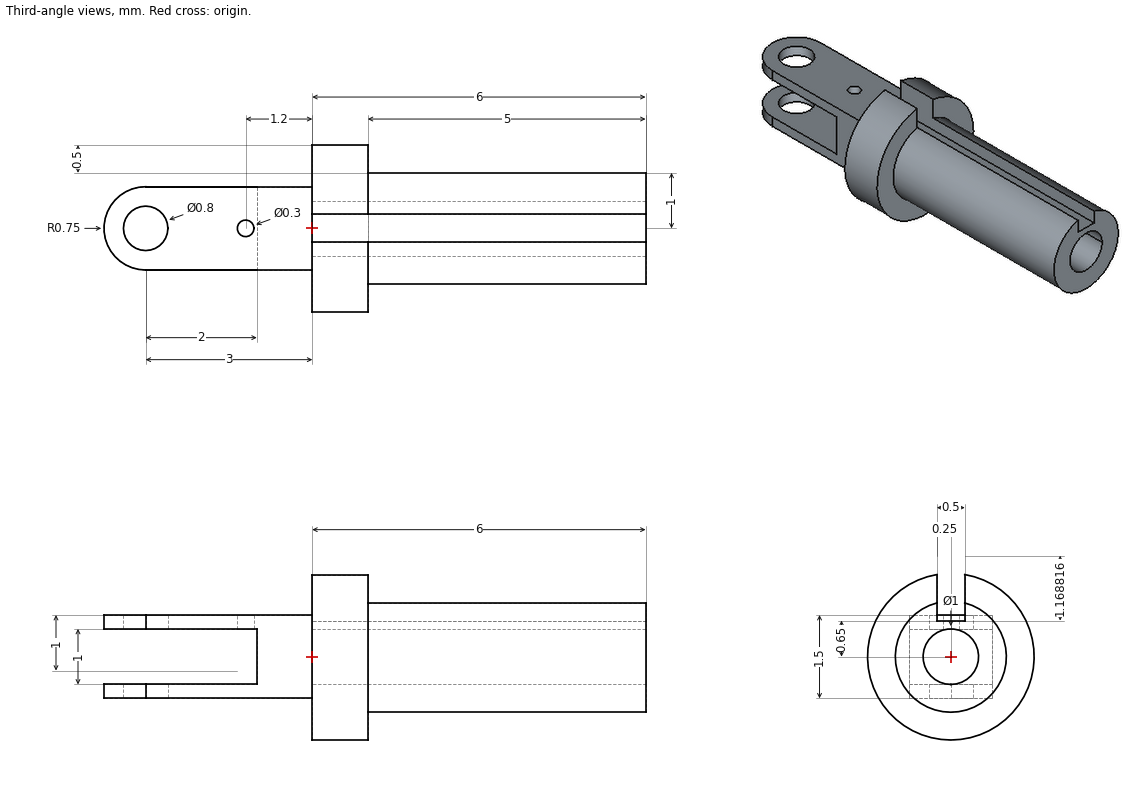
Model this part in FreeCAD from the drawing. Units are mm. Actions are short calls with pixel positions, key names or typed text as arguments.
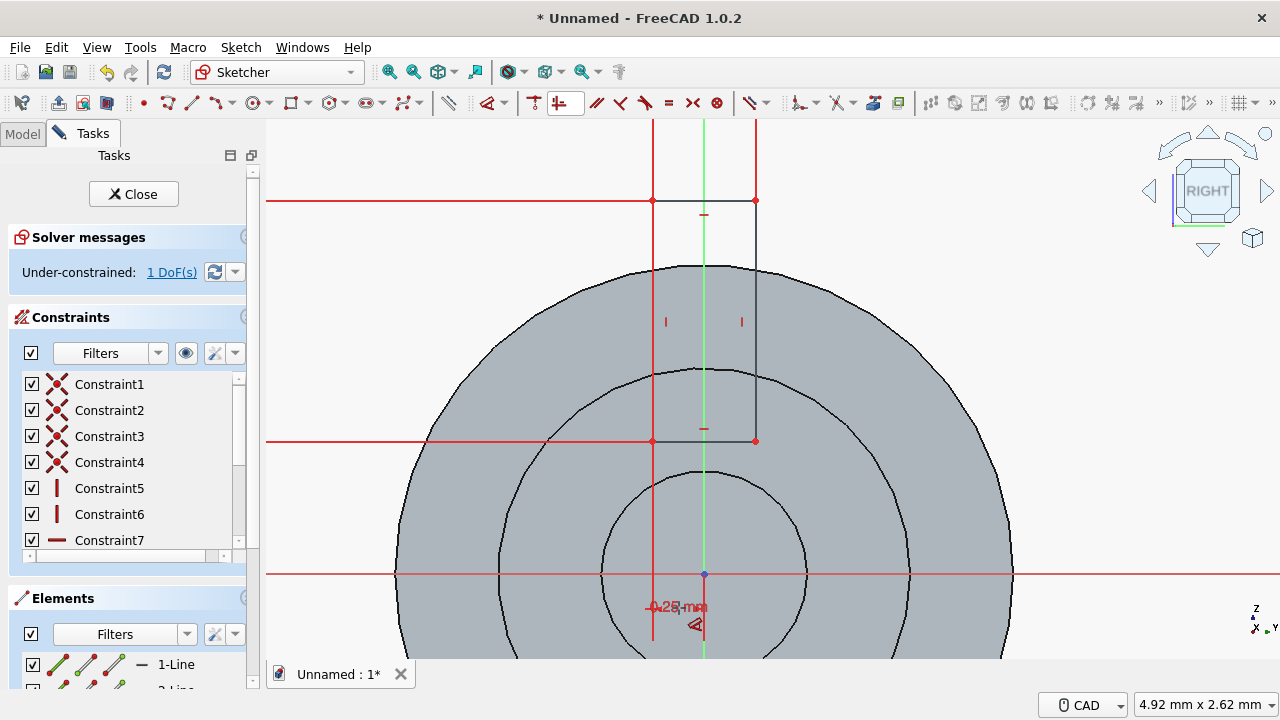
click(653, 442)
click(619, 508)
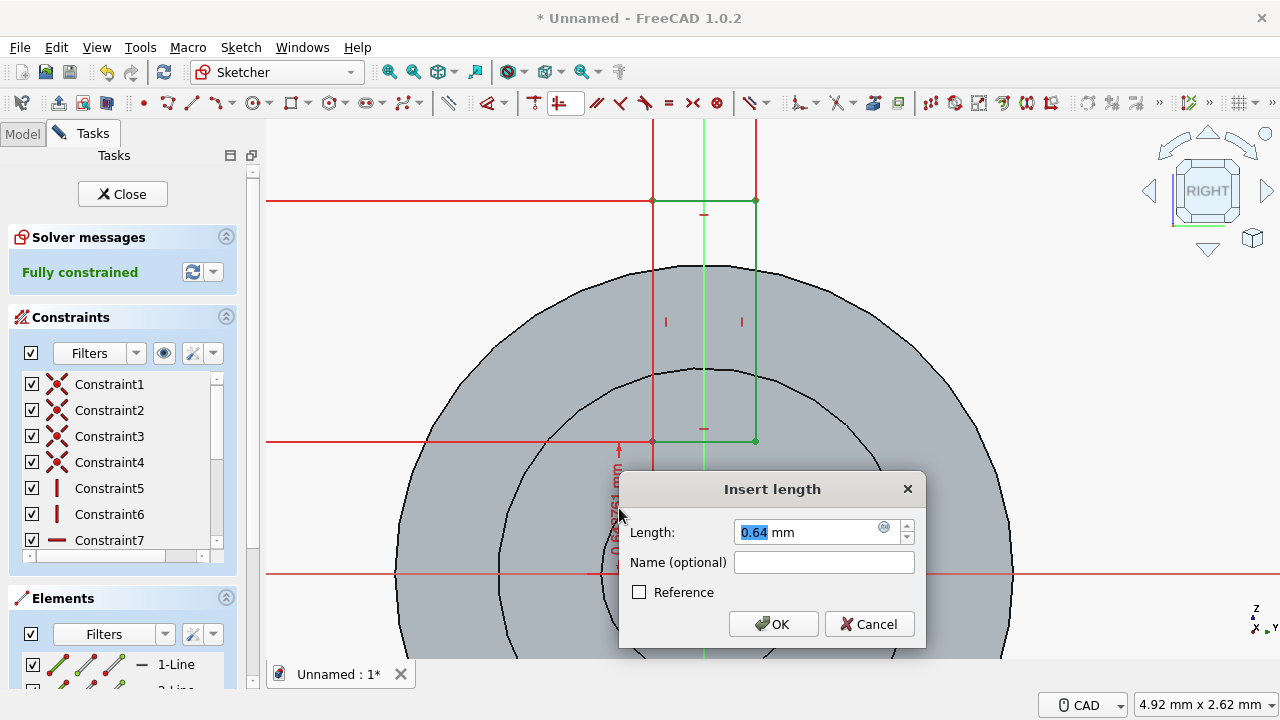
text(0.65)
key(Return)
key(Escape)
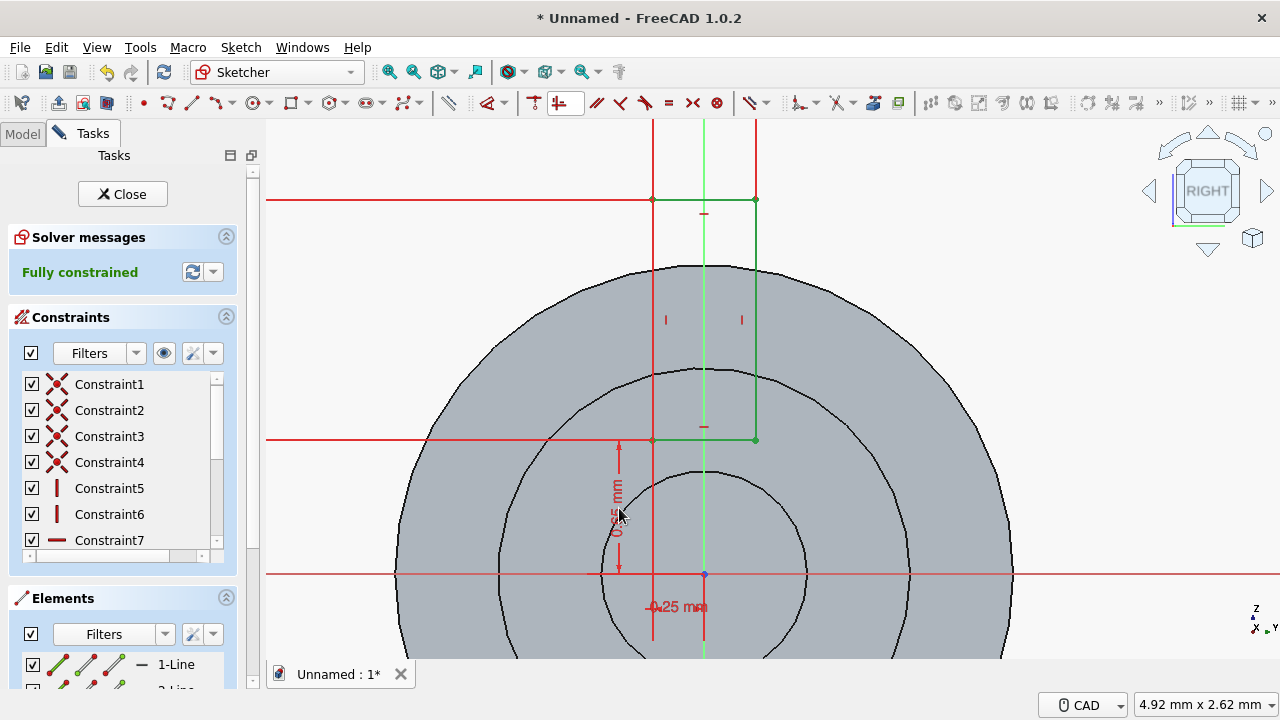
click(123, 194)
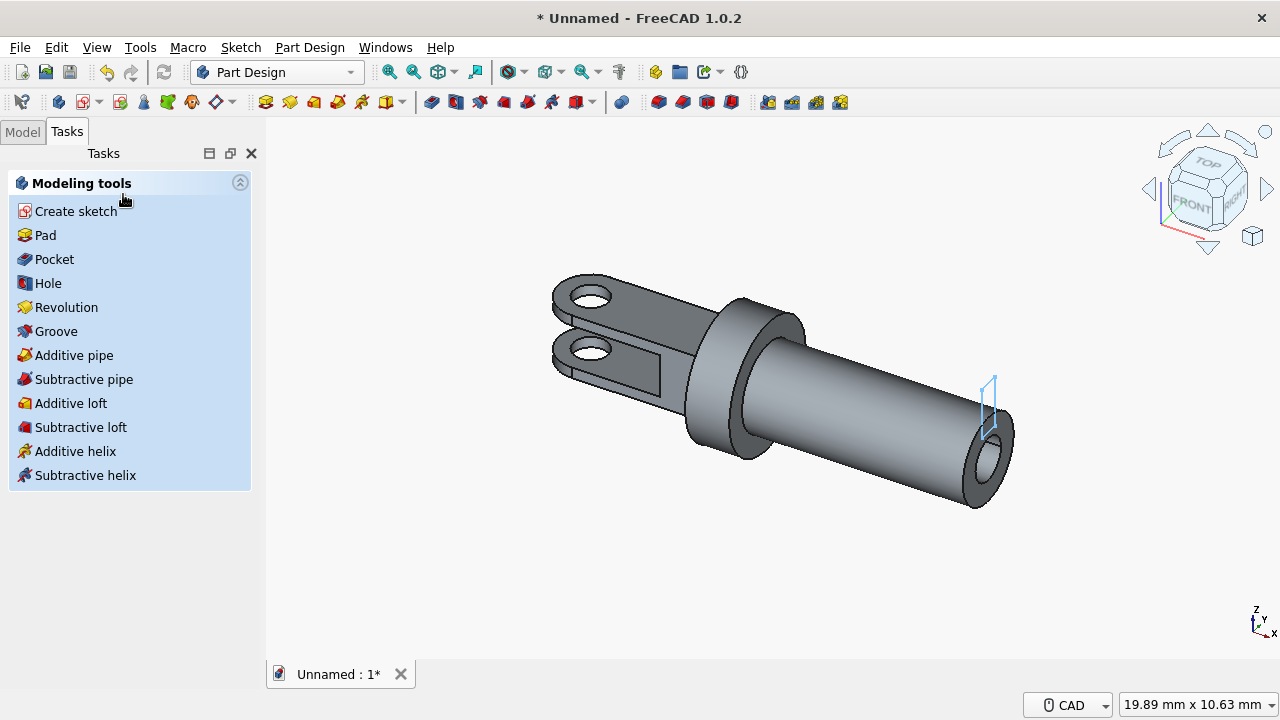
click(432, 102)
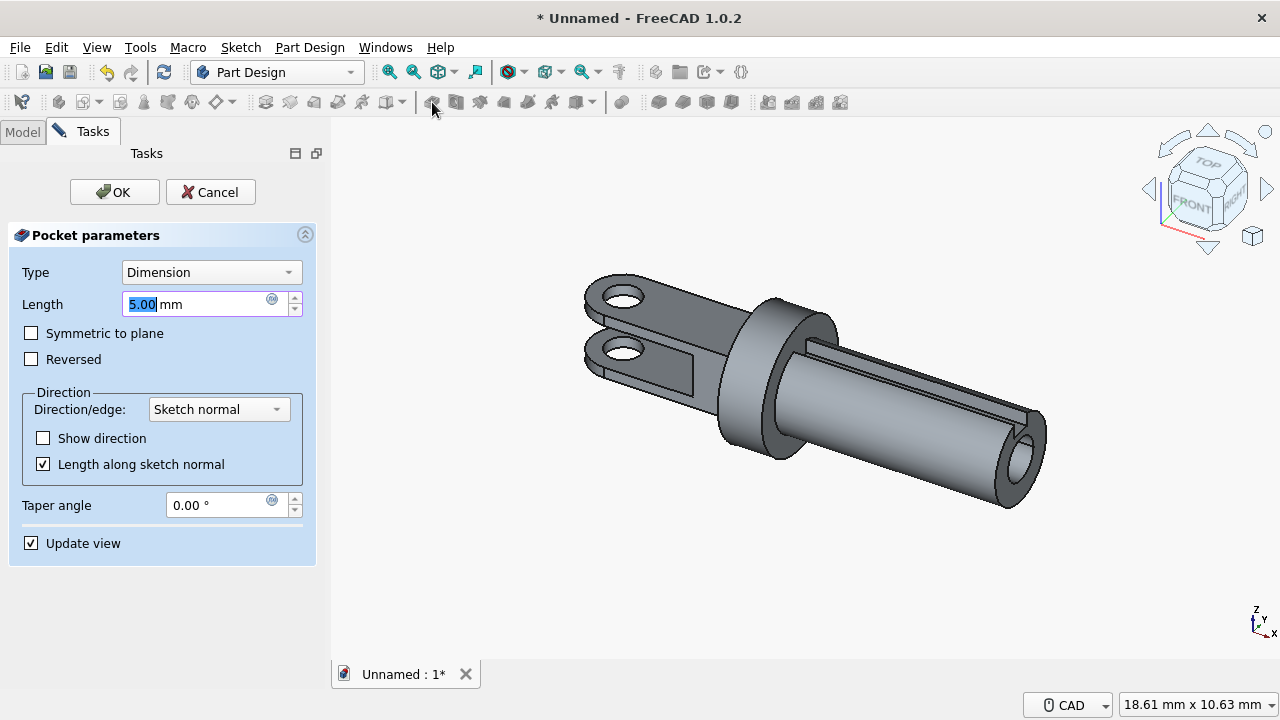
text(6)
key(Tab)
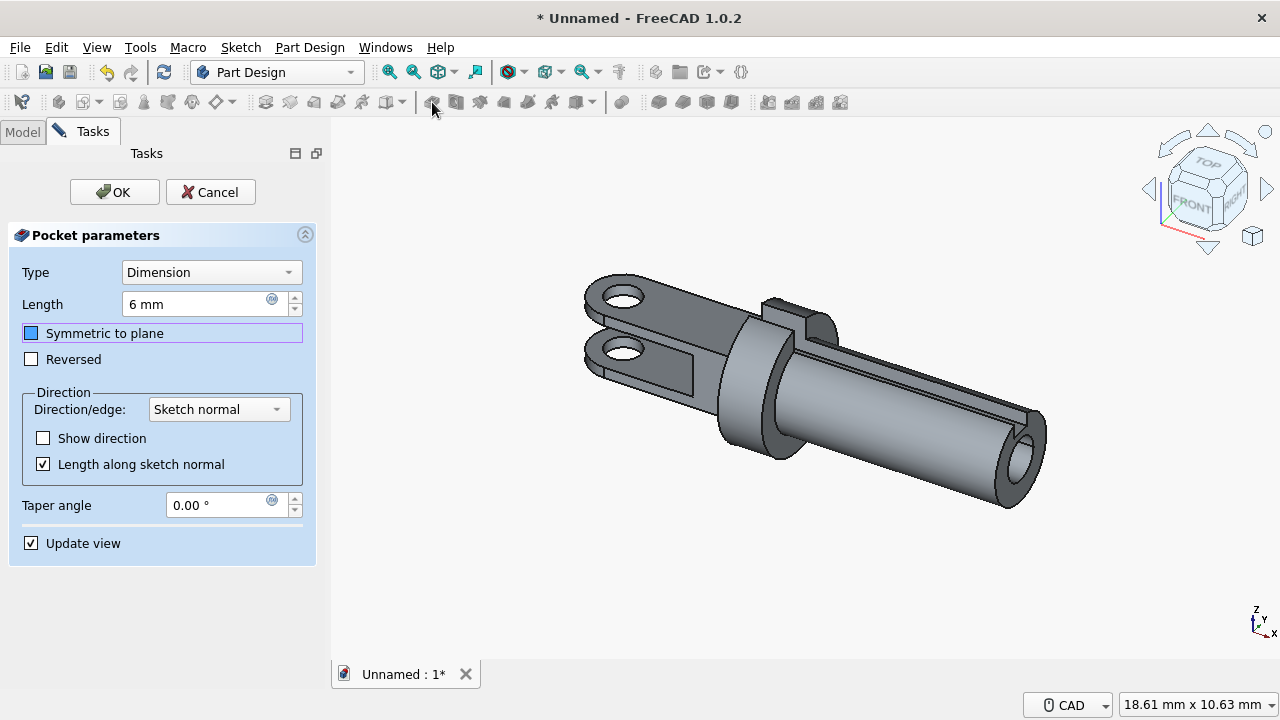
click(115, 192)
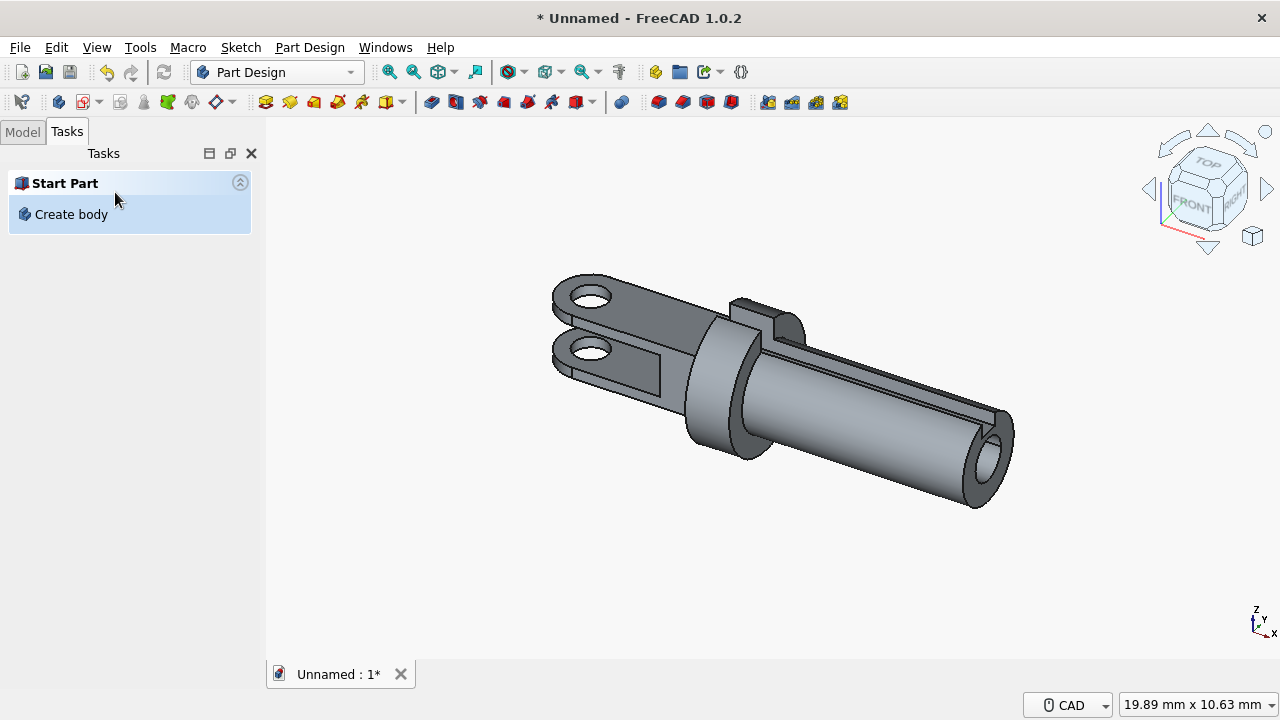
key(0)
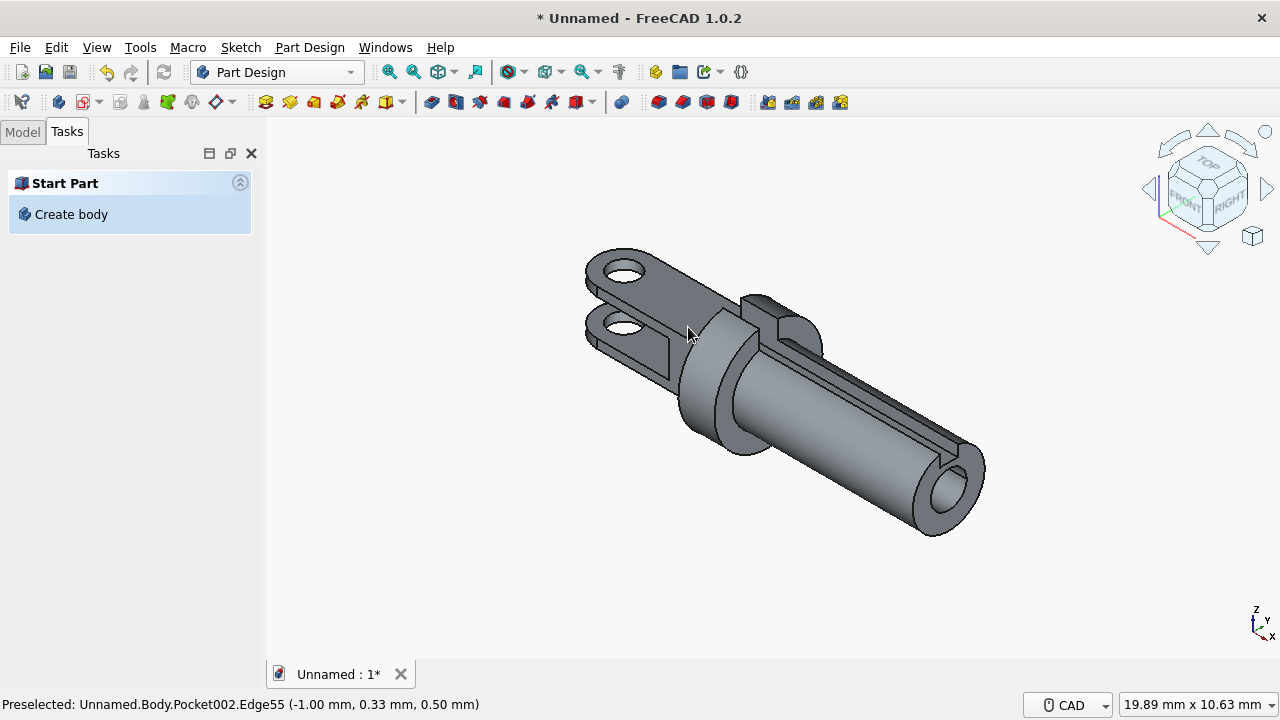
click(684, 304)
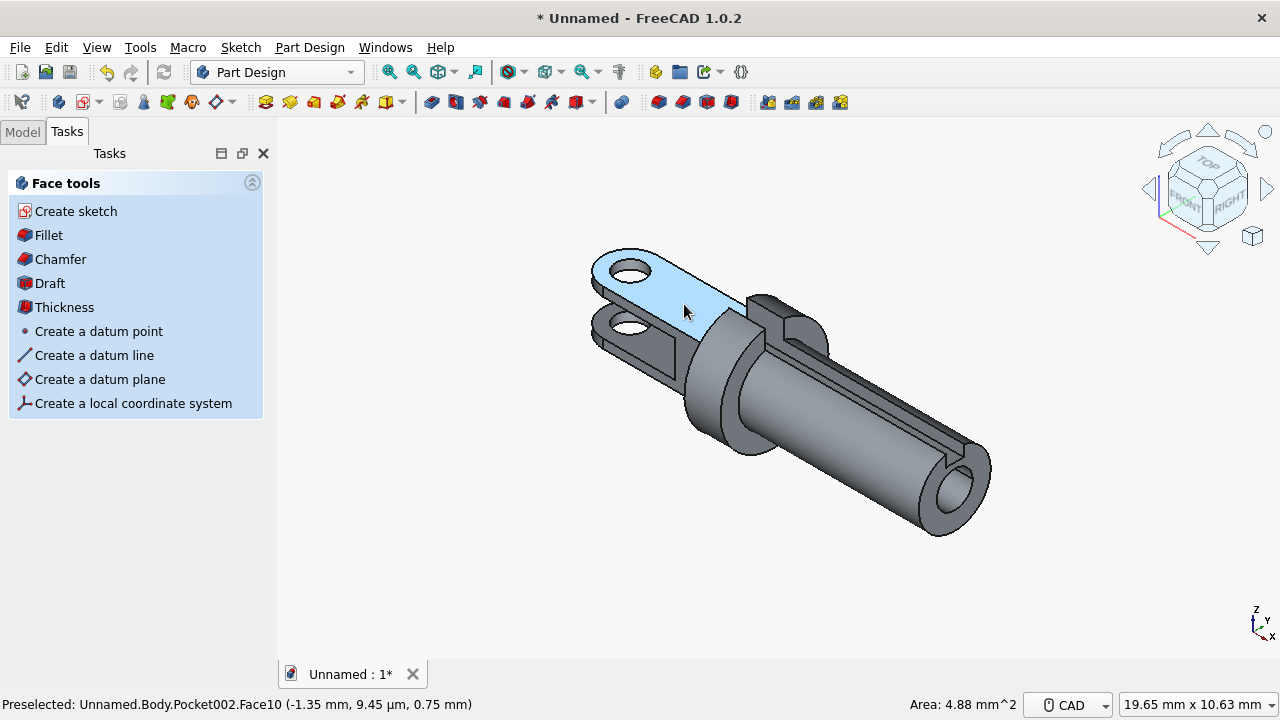
click(84, 102)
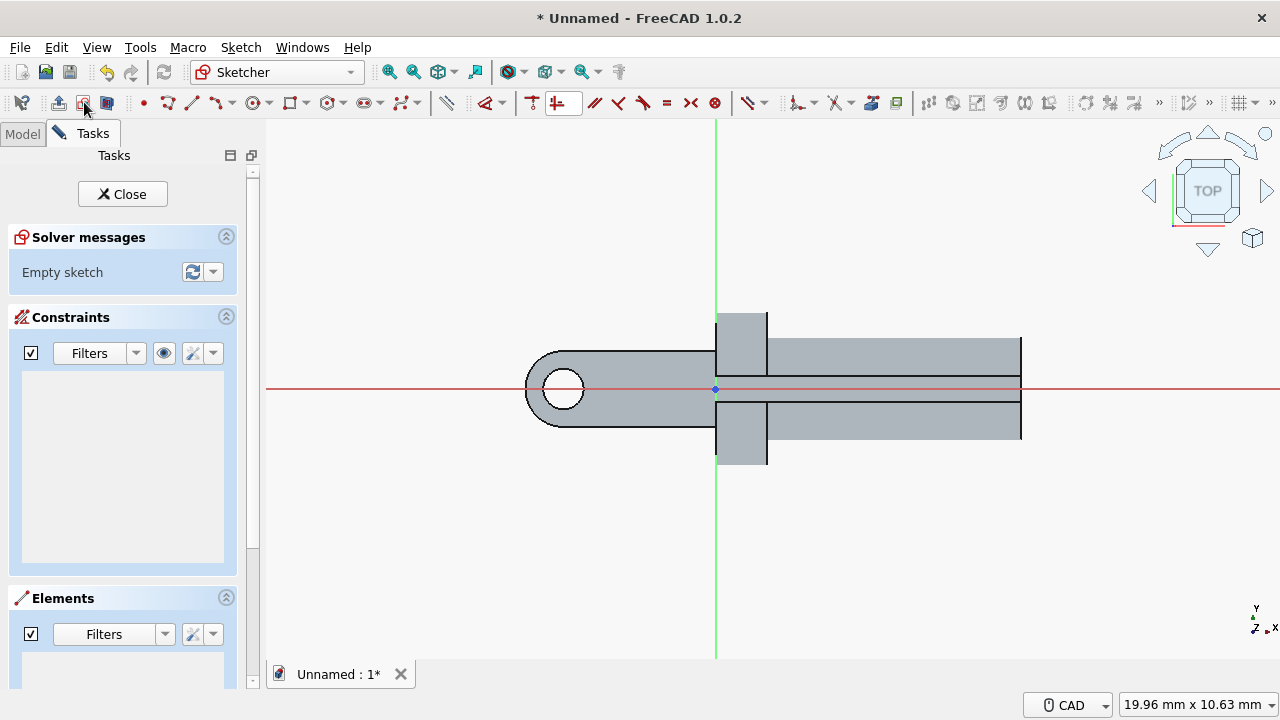
click(108, 104)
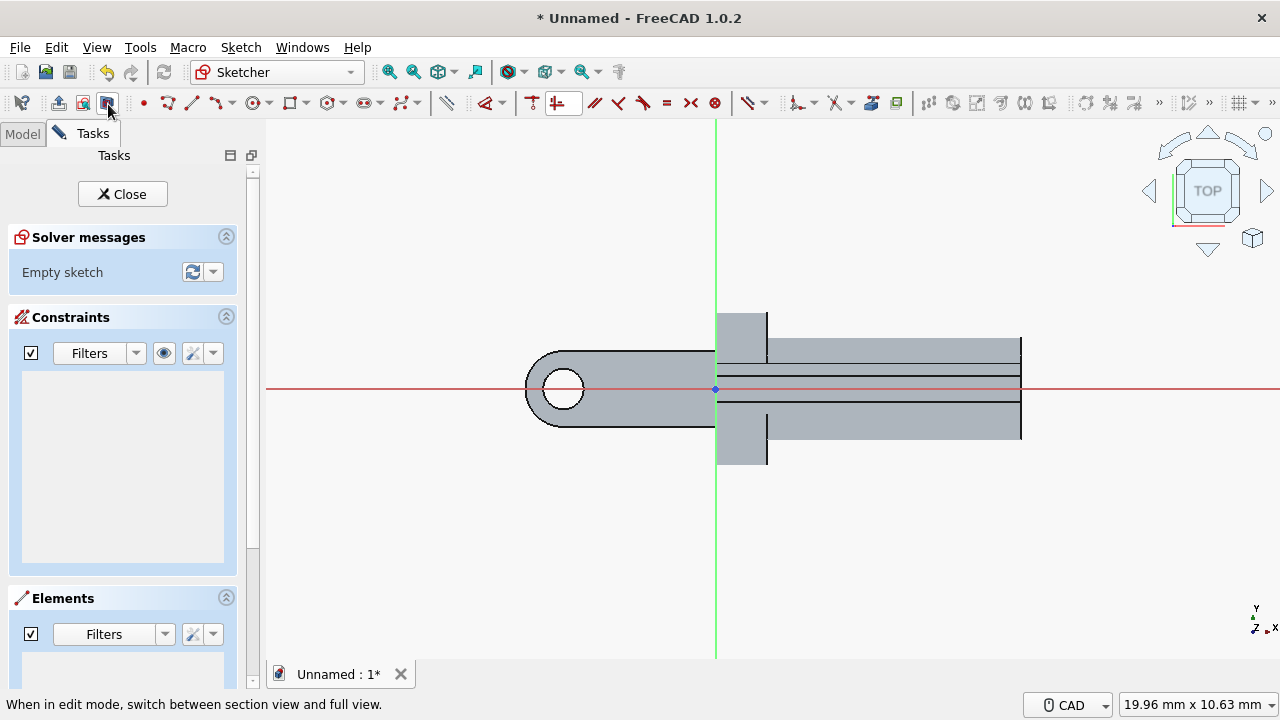
scroll(652, 389, up, 15)